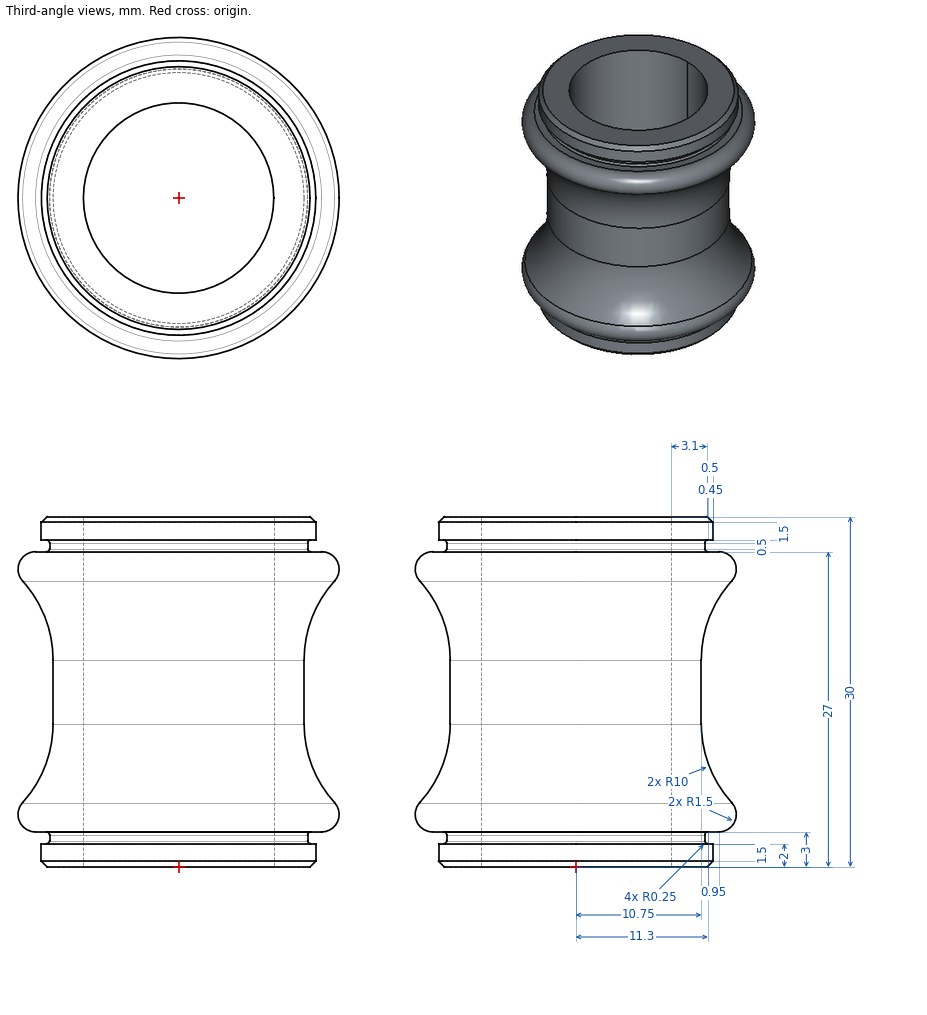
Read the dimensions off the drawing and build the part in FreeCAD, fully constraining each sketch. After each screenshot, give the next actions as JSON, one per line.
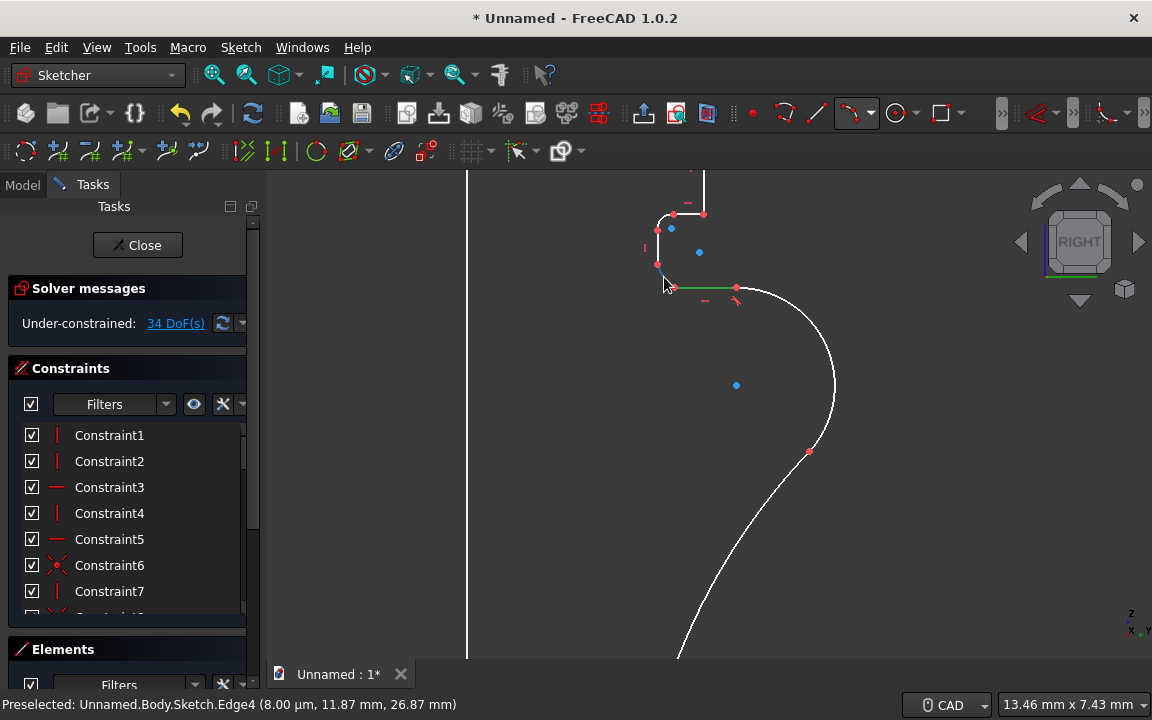
{"action": "left_click", "coordinate": [664, 277]}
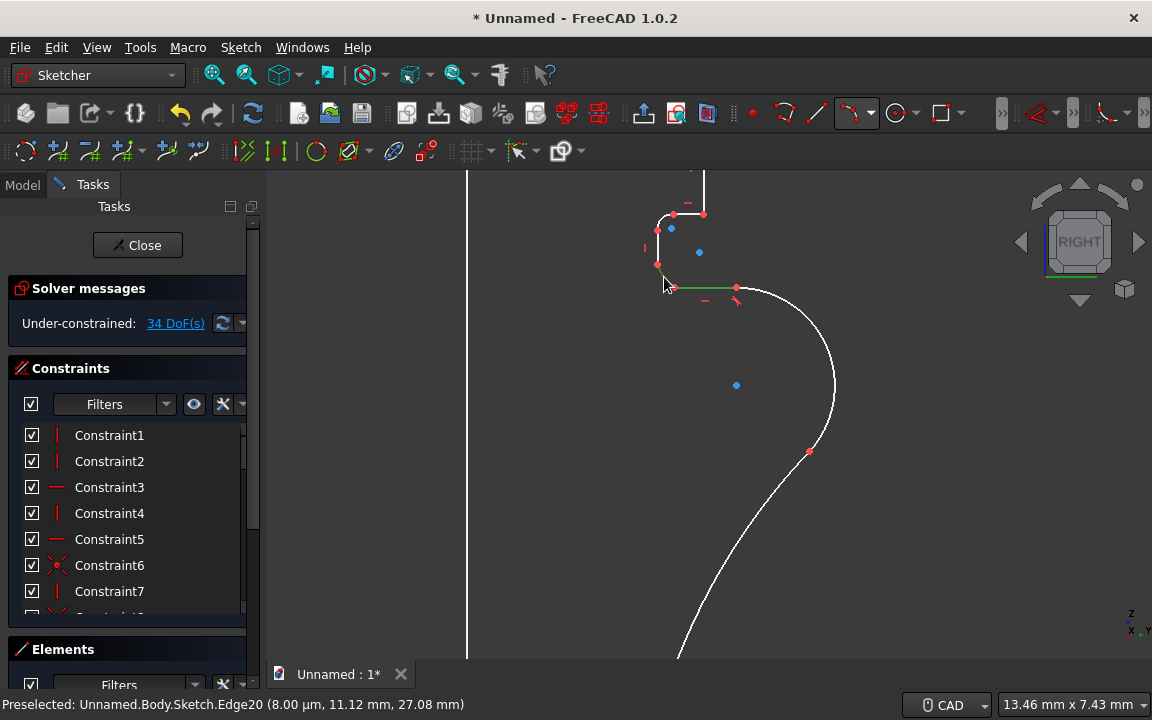
{"action": "key", "text": "t"}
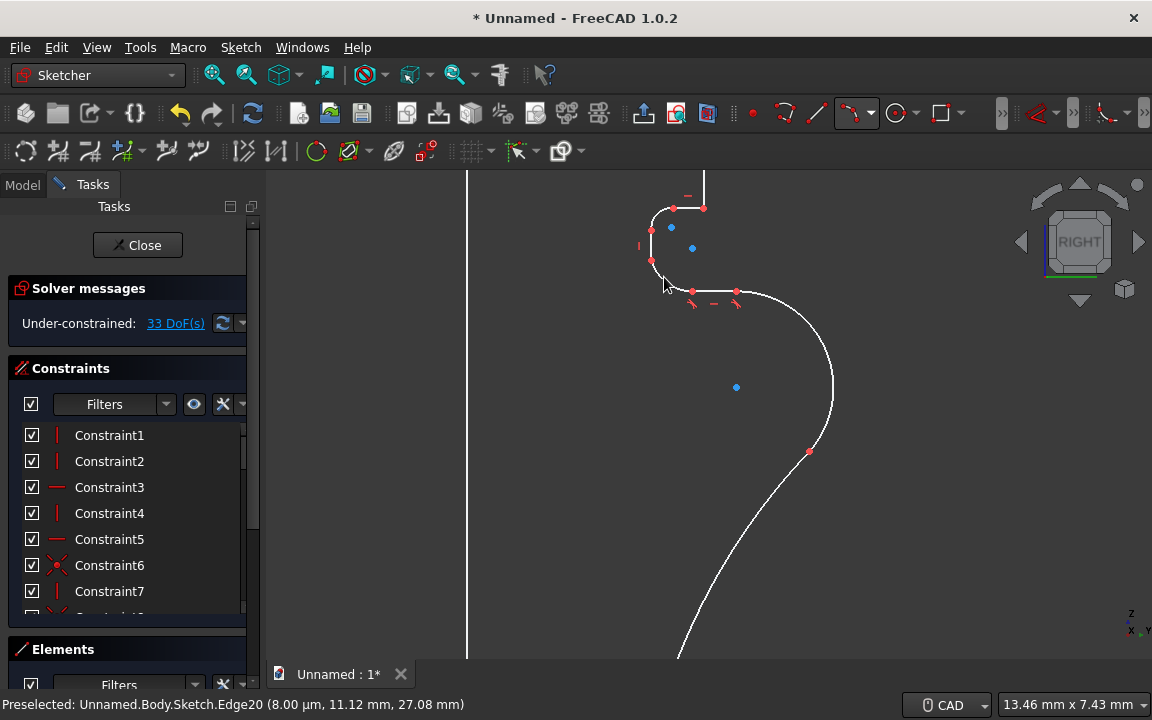
{"action": "scroll", "coordinate": [651, 251], "scroll_direction": "up", "scroll_amount": 3}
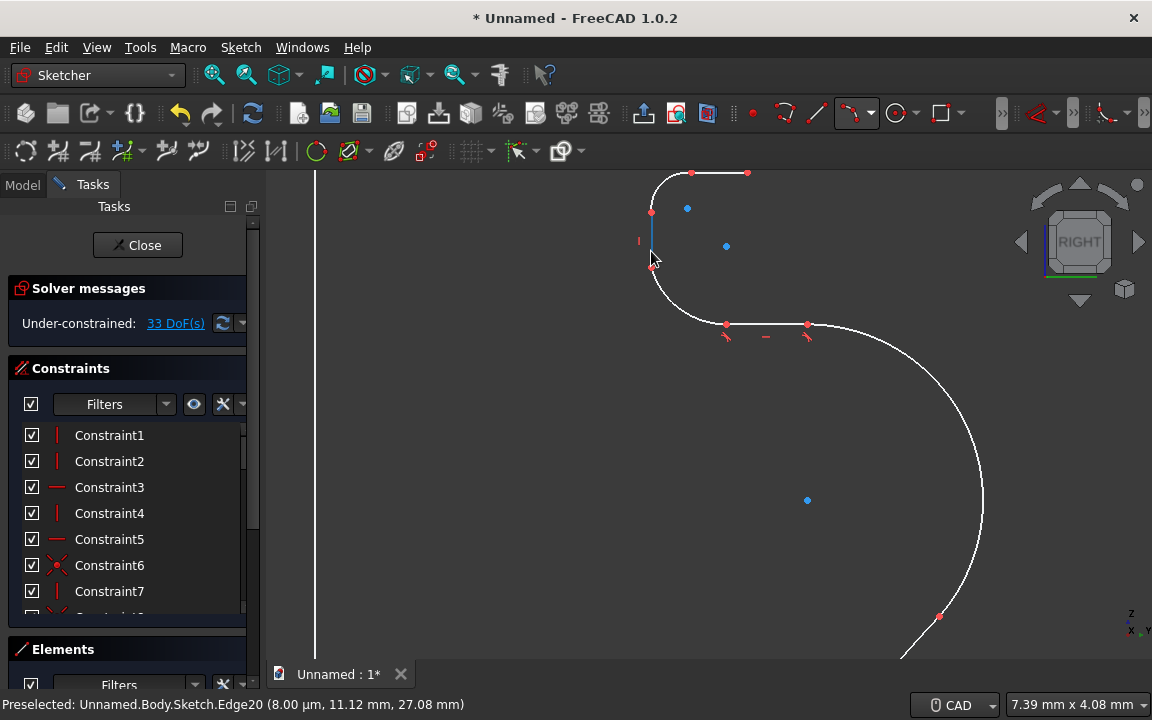
{"action": "left_click", "coordinate": [652, 251]}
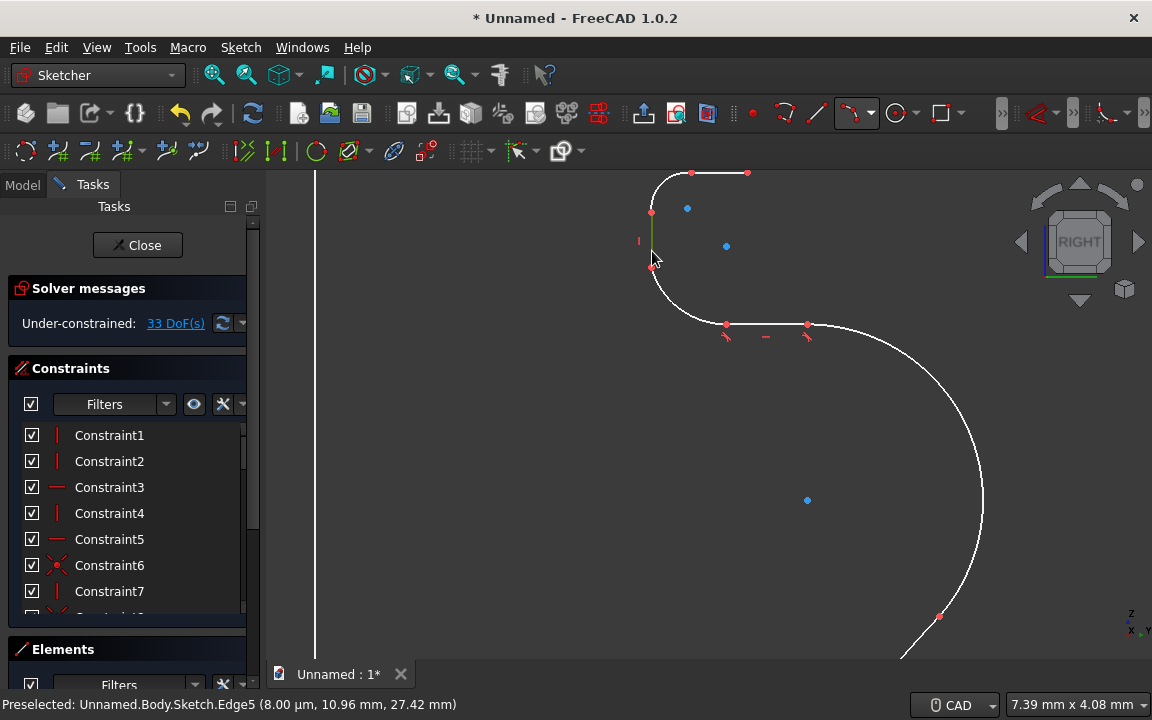
{"action": "left_click", "coordinate": [665, 295]}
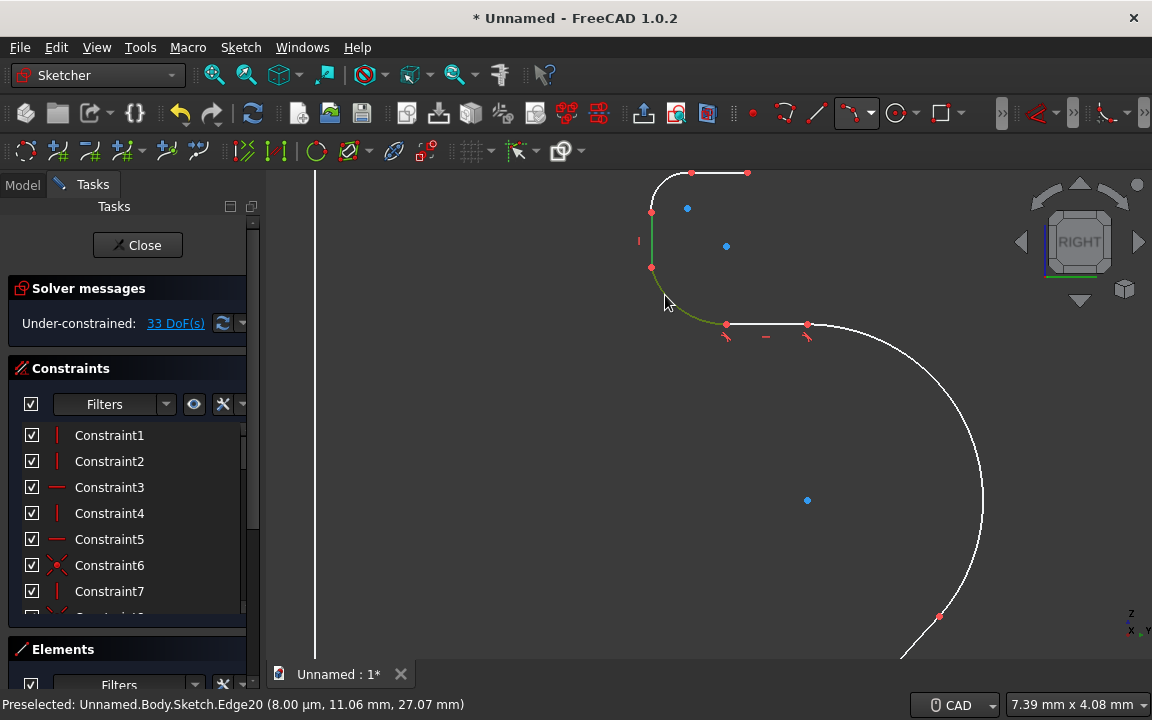
{"action": "key", "text": "t"}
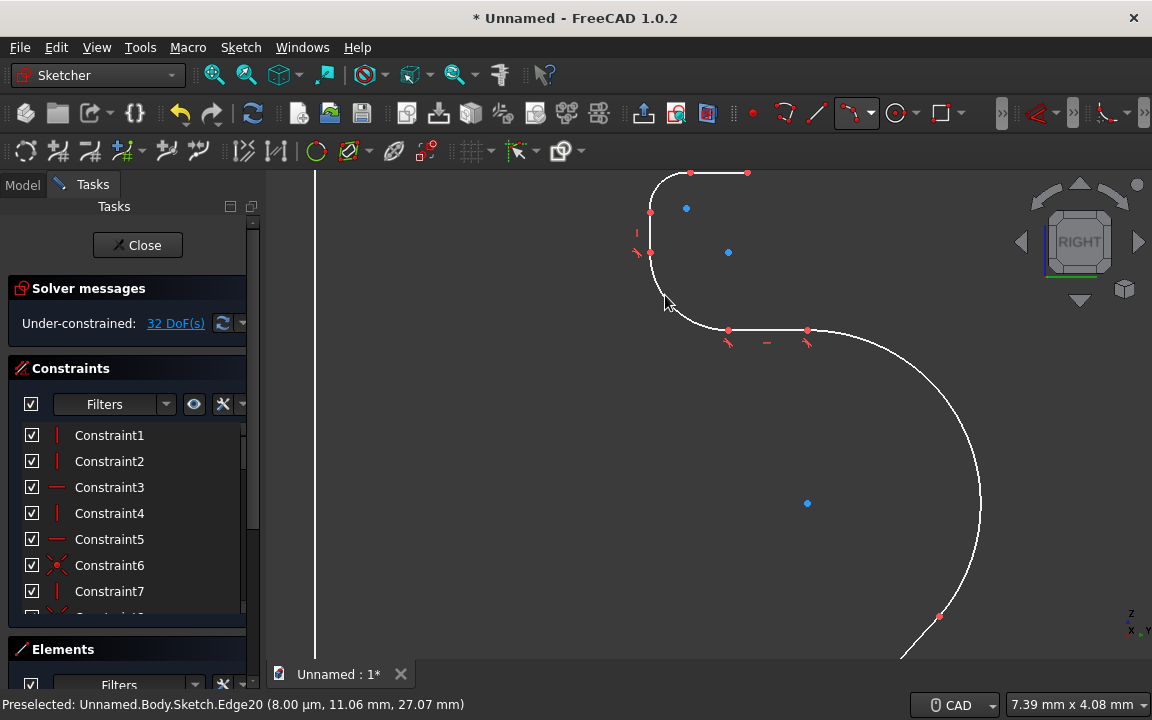
{"action": "left_click", "coordinate": [650, 240]}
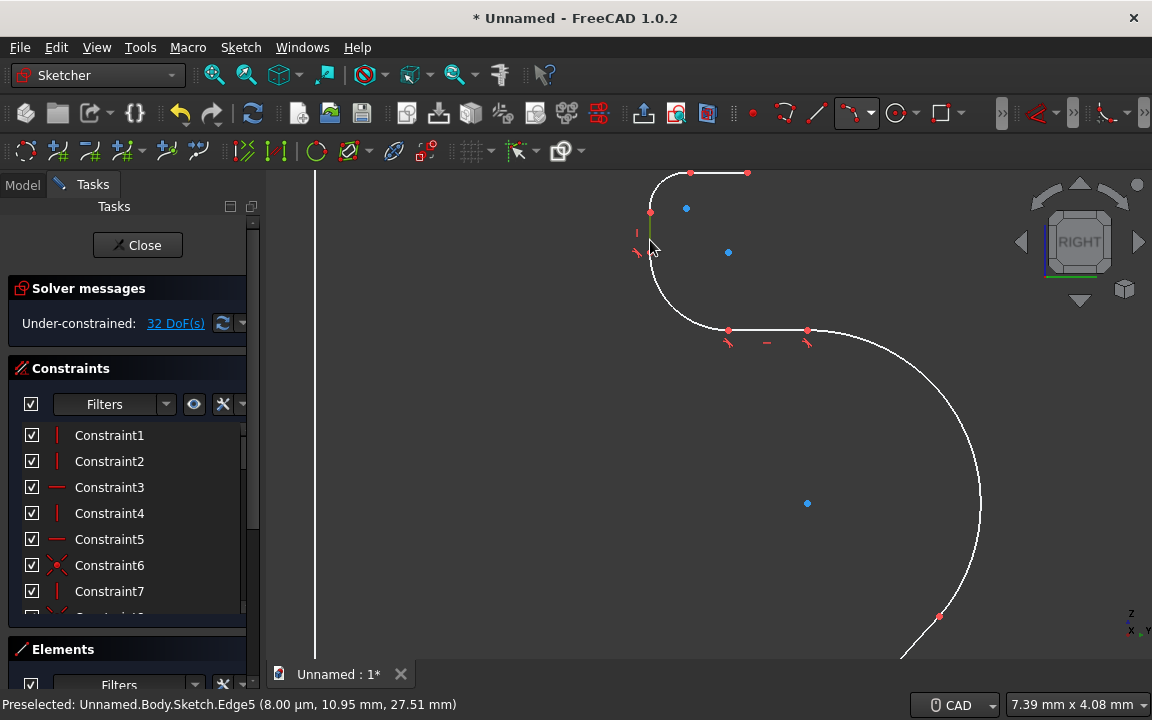
{"action": "left_click", "coordinate": [651, 200]}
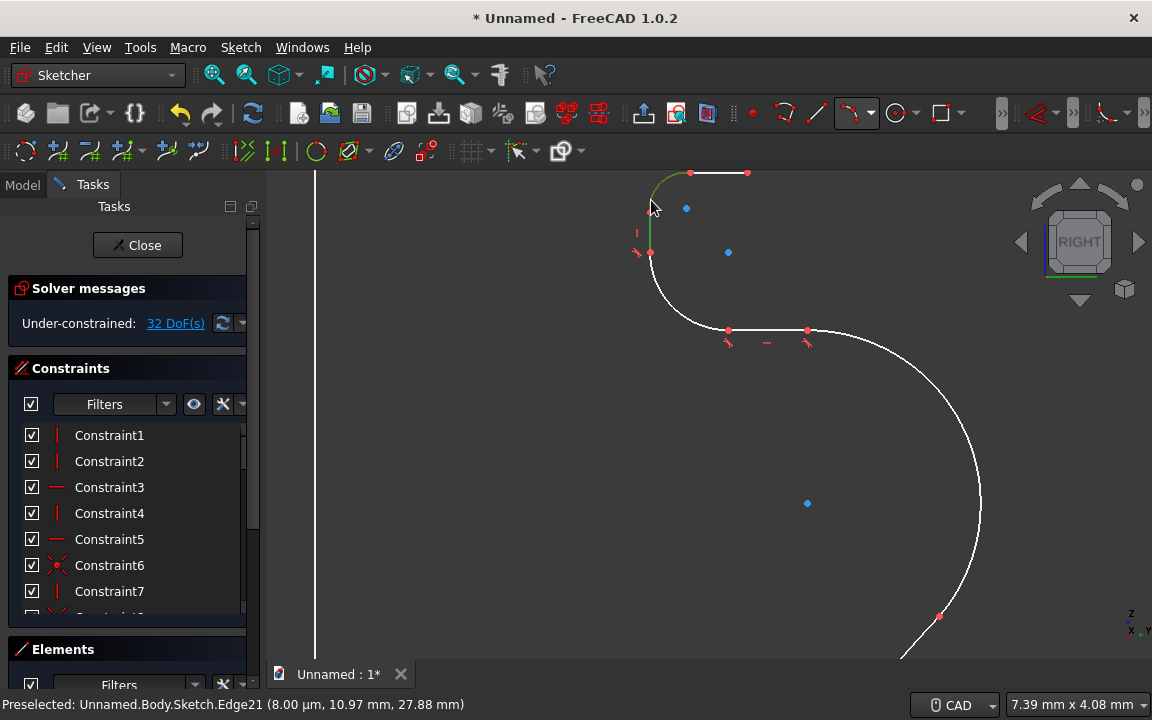
{"action": "key", "text": "t"}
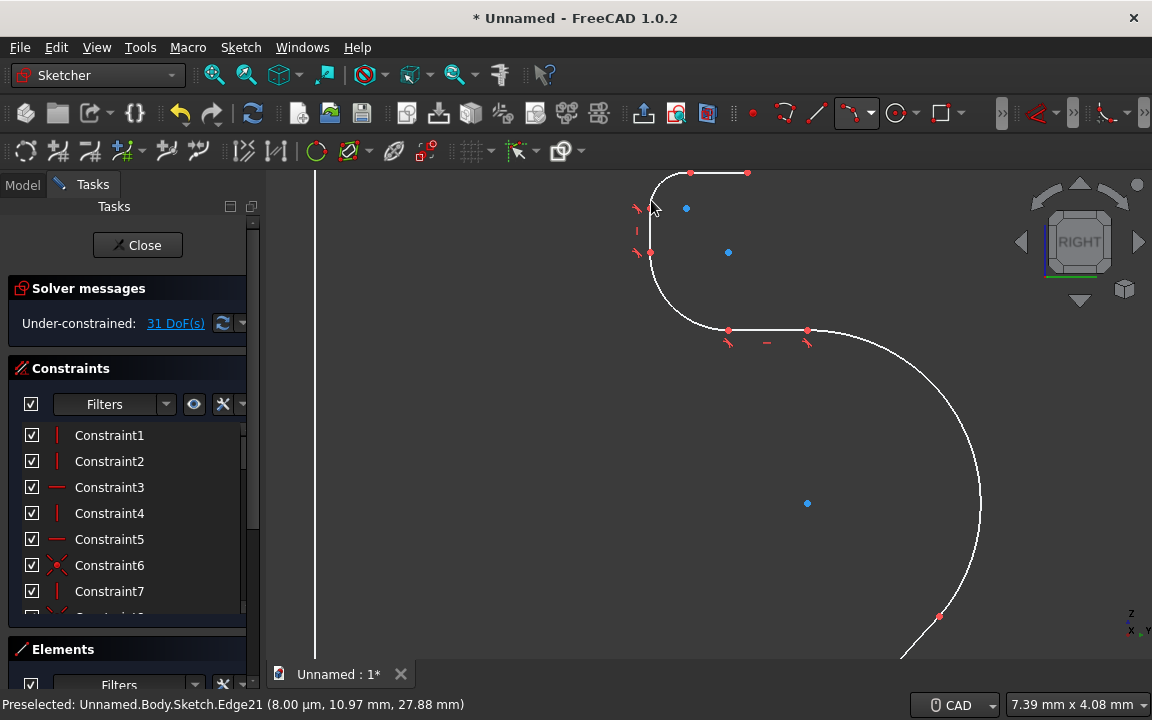
{"action": "scroll", "coordinate": [689, 282], "scroll_direction": "down", "scroll_amount": 12}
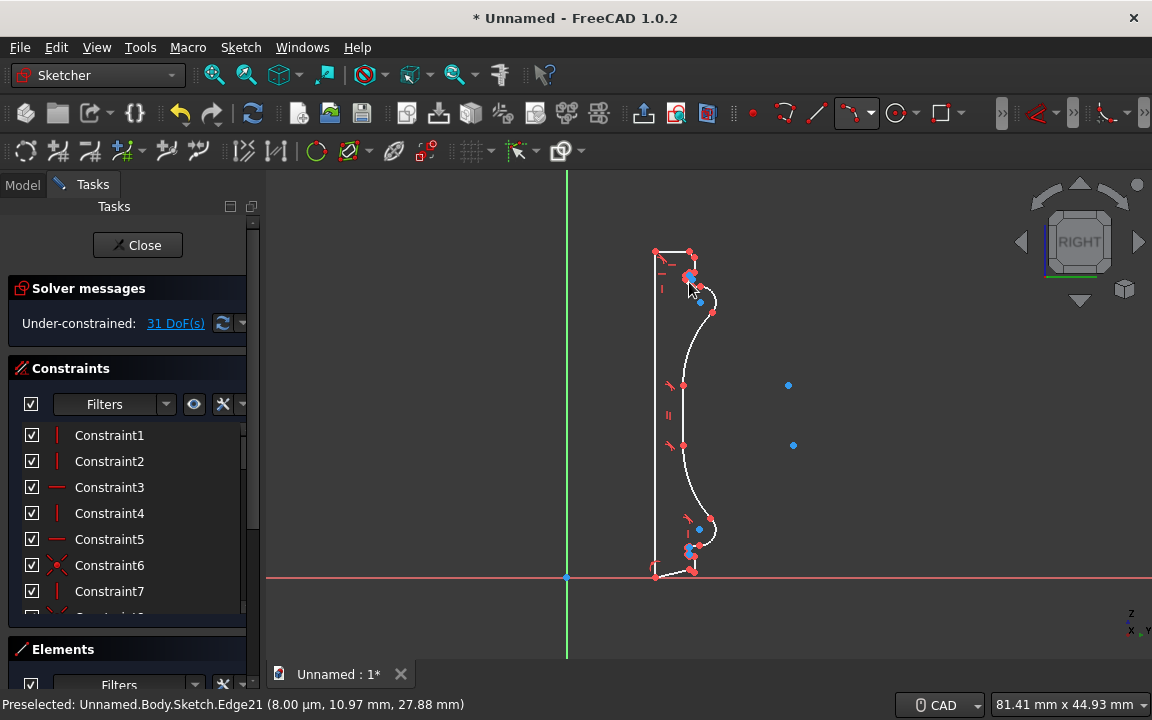
{"action": "scroll", "coordinate": [691, 272], "scroll_direction": "up", "scroll_amount": 11}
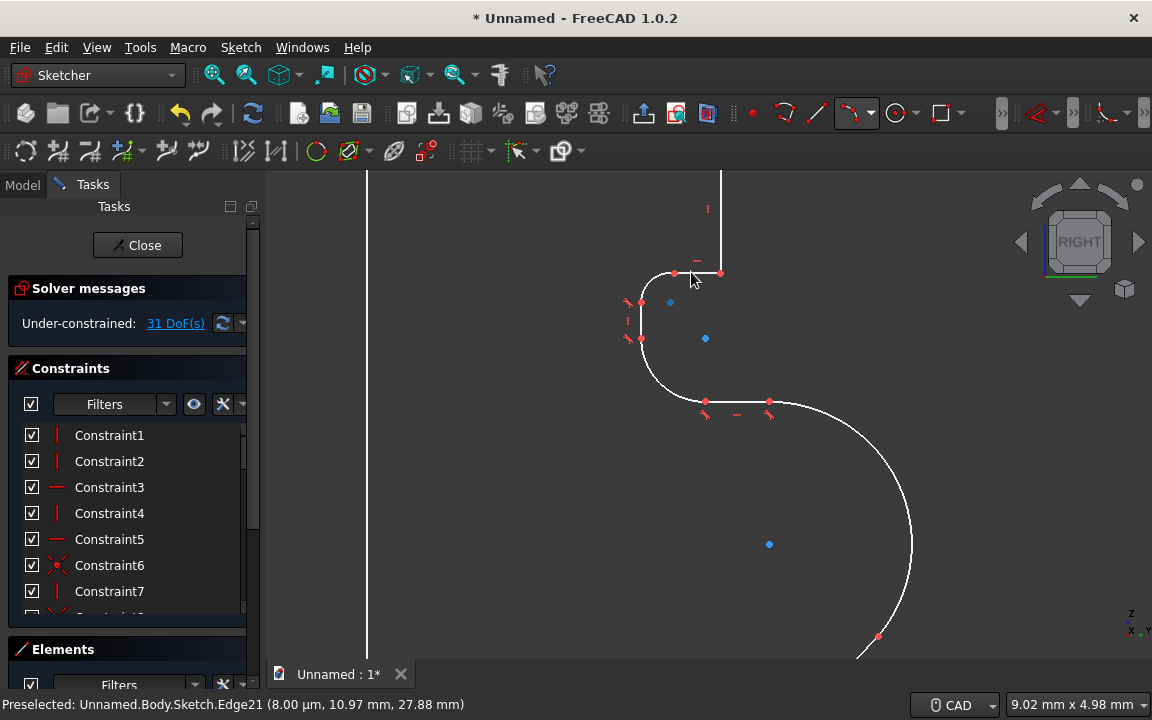
{"action": "left_click", "coordinate": [688, 273]}